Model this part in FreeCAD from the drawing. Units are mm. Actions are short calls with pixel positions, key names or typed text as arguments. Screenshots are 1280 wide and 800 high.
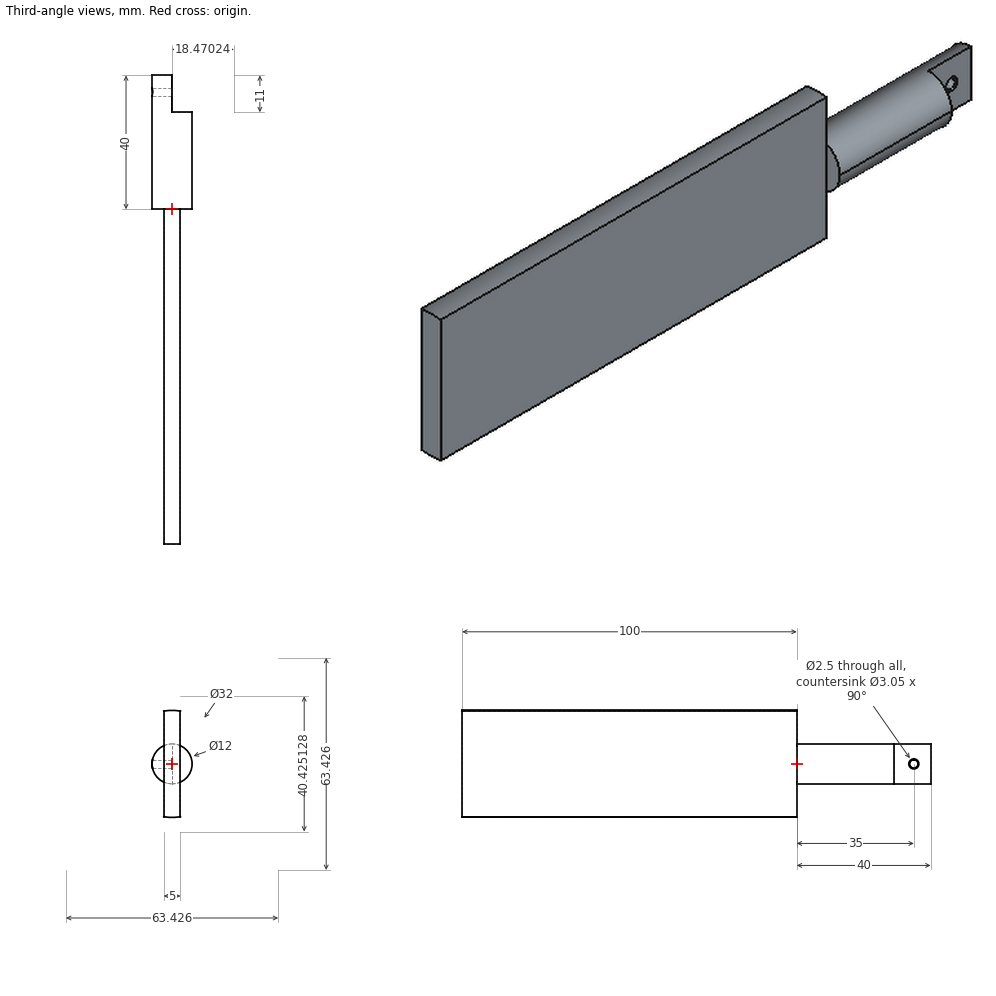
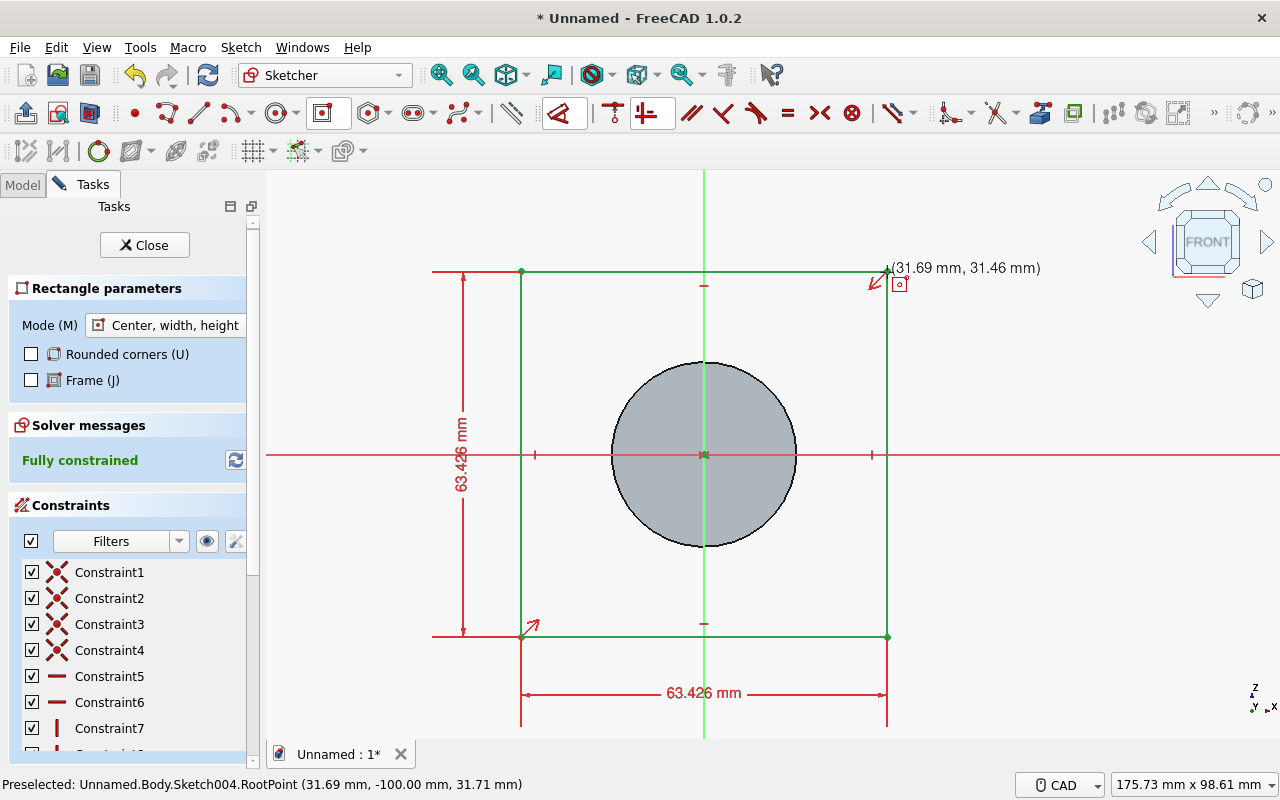
click(704, 454)
move(719, 338)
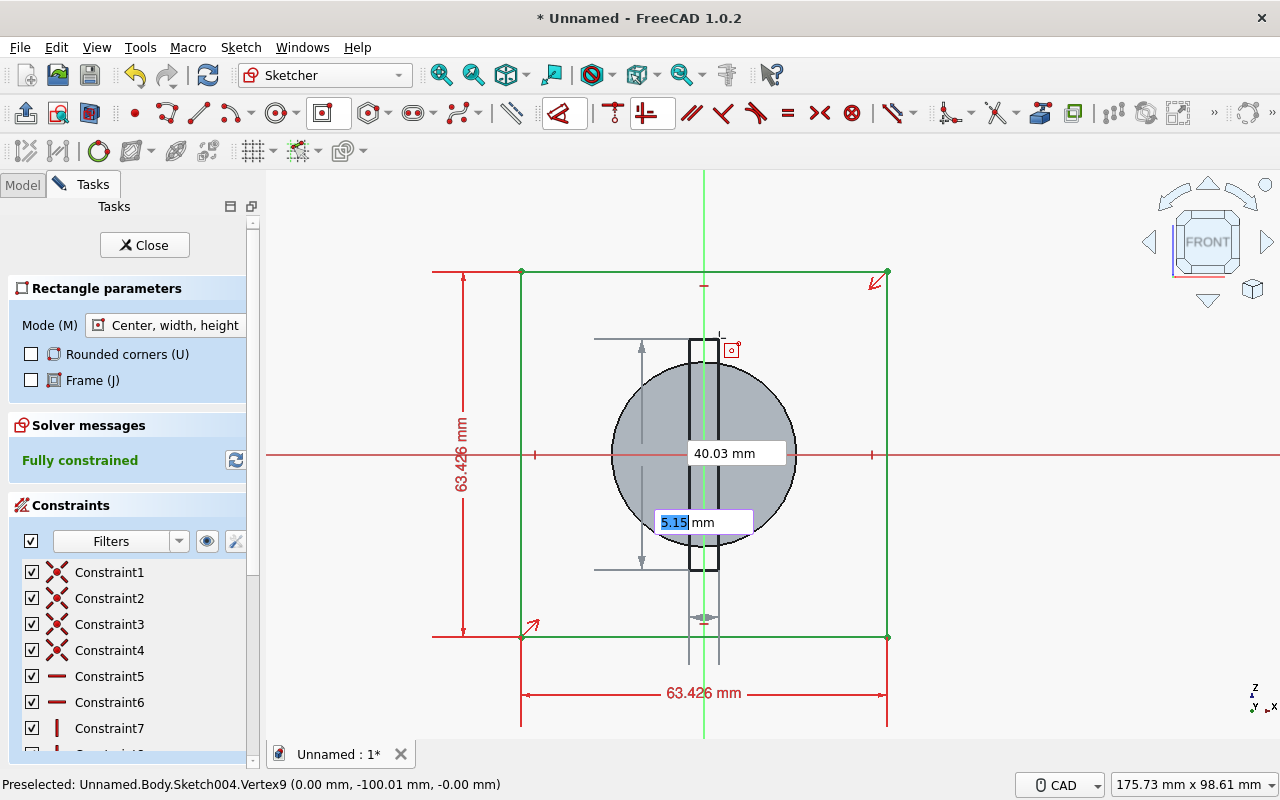
text(5)
key(Tab)
text(40.425128)
key(Return)
key(Escape)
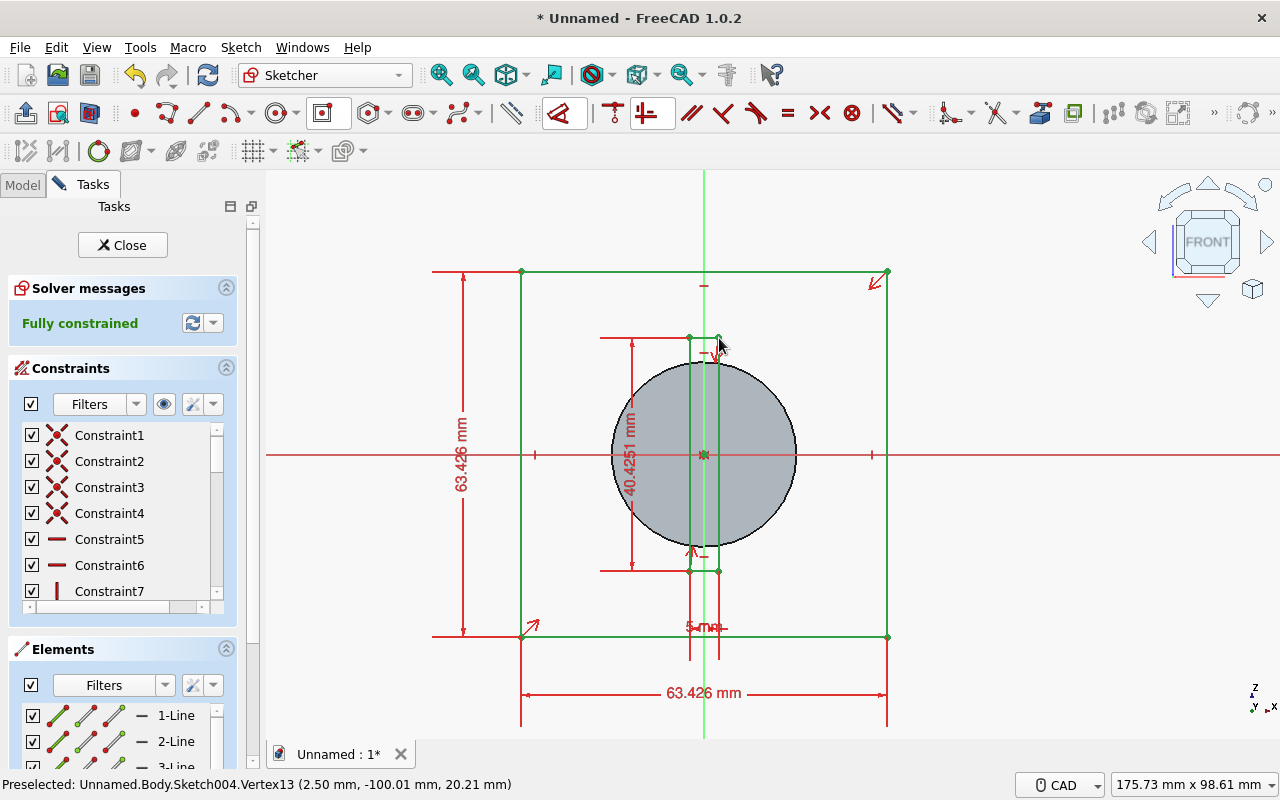
click(123, 245)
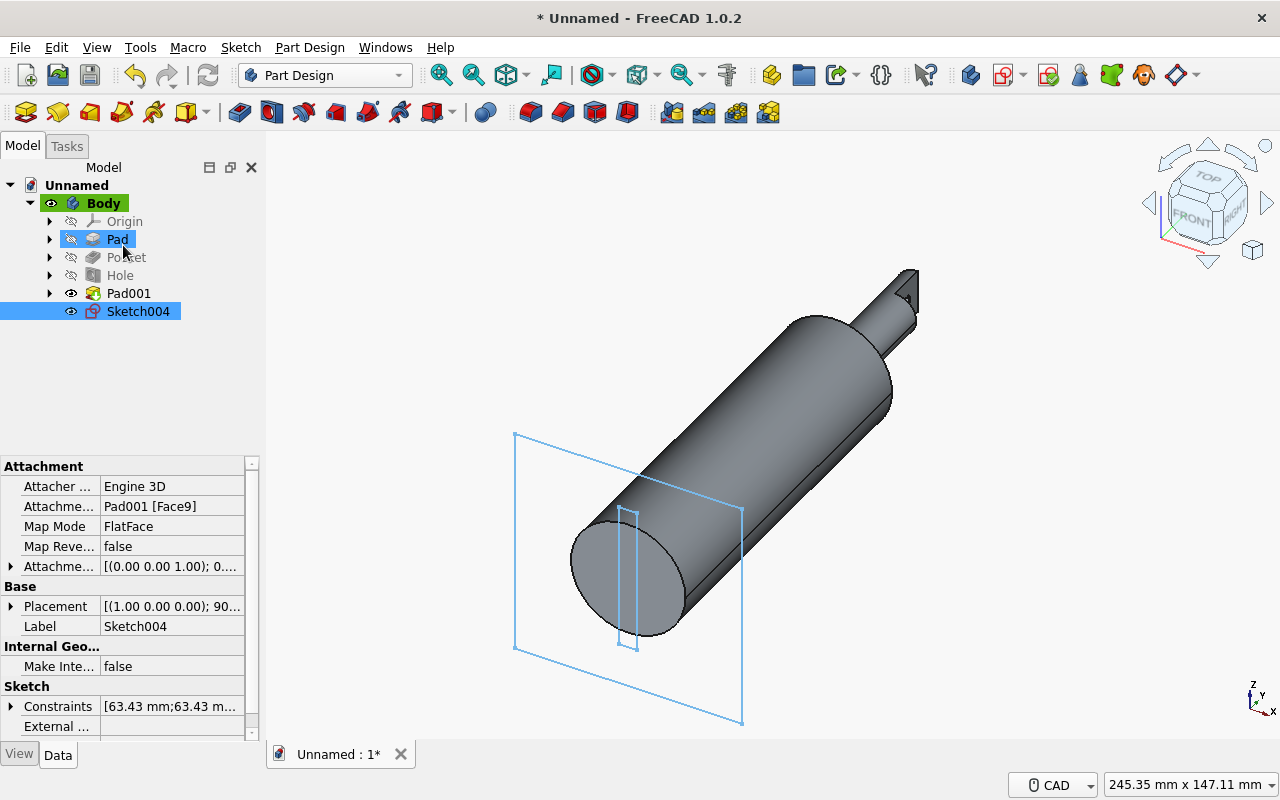
click(240, 112)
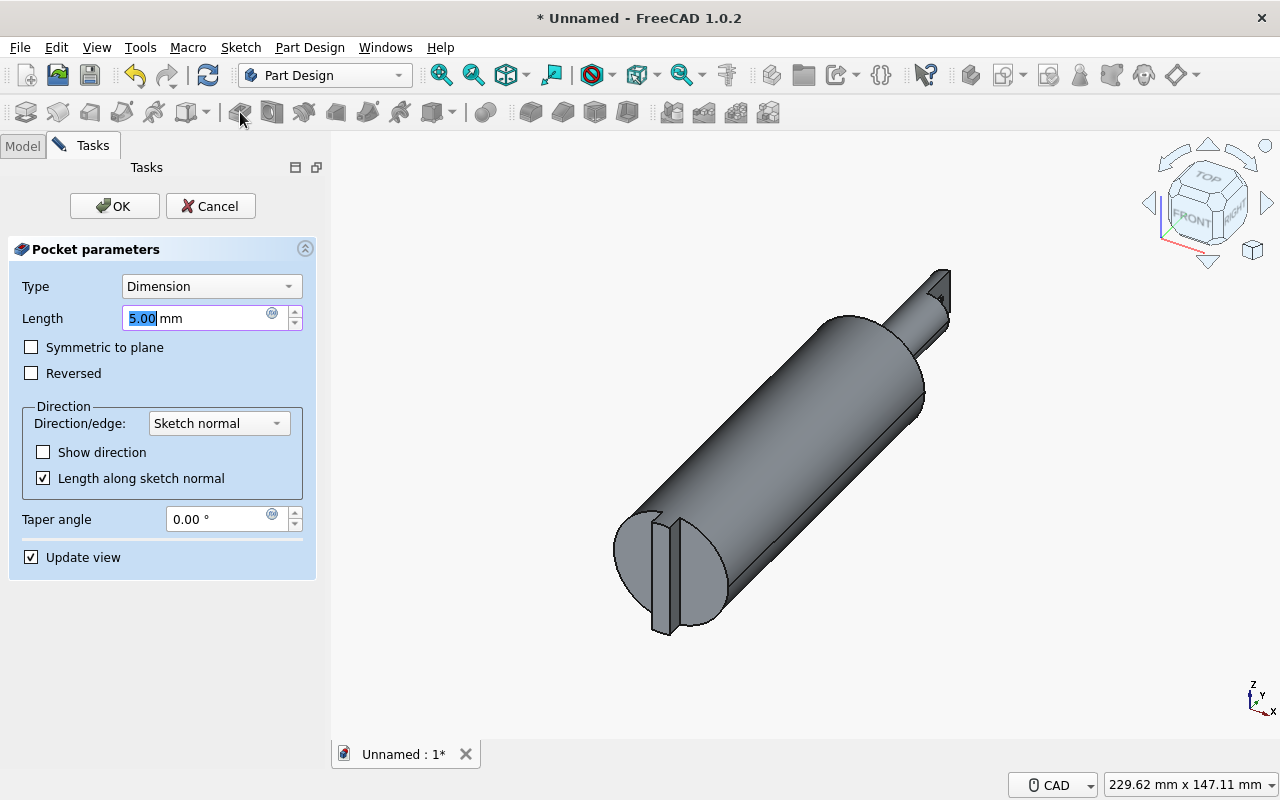
click(212, 286)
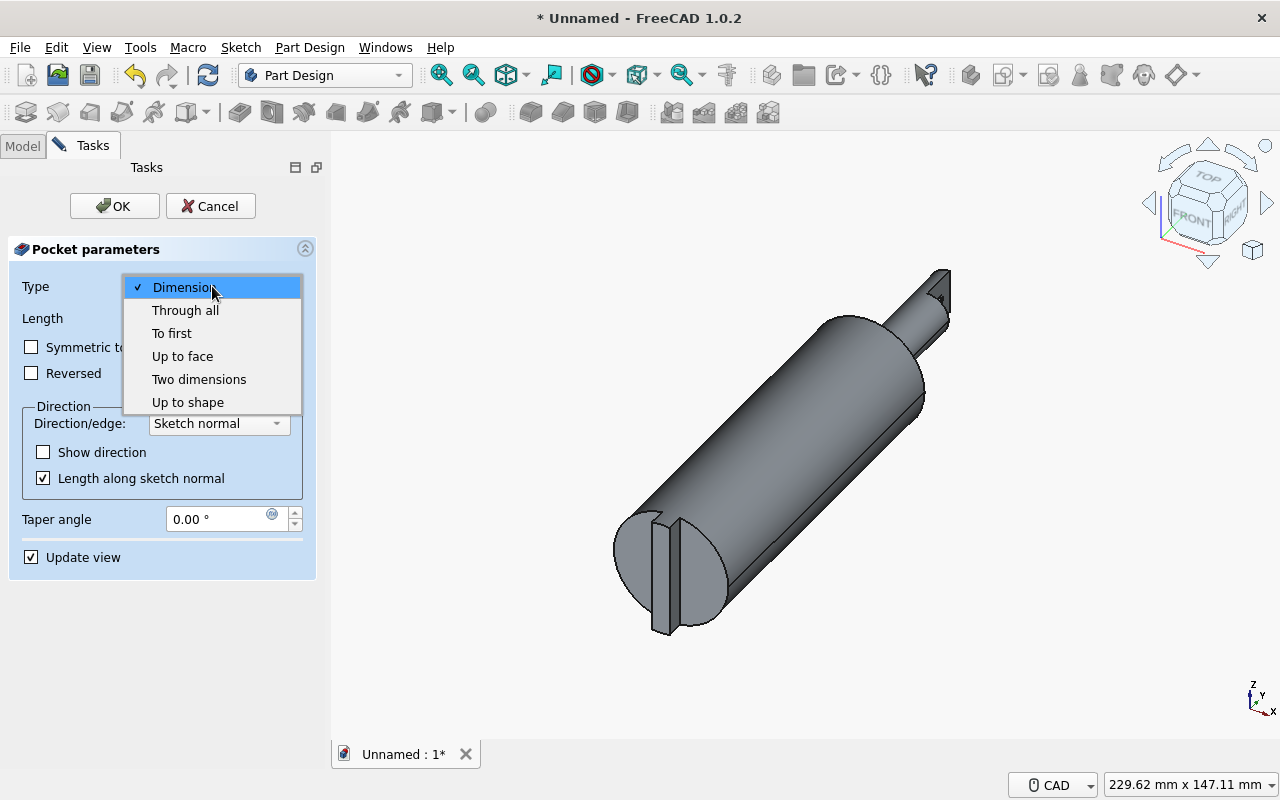
click(212, 380)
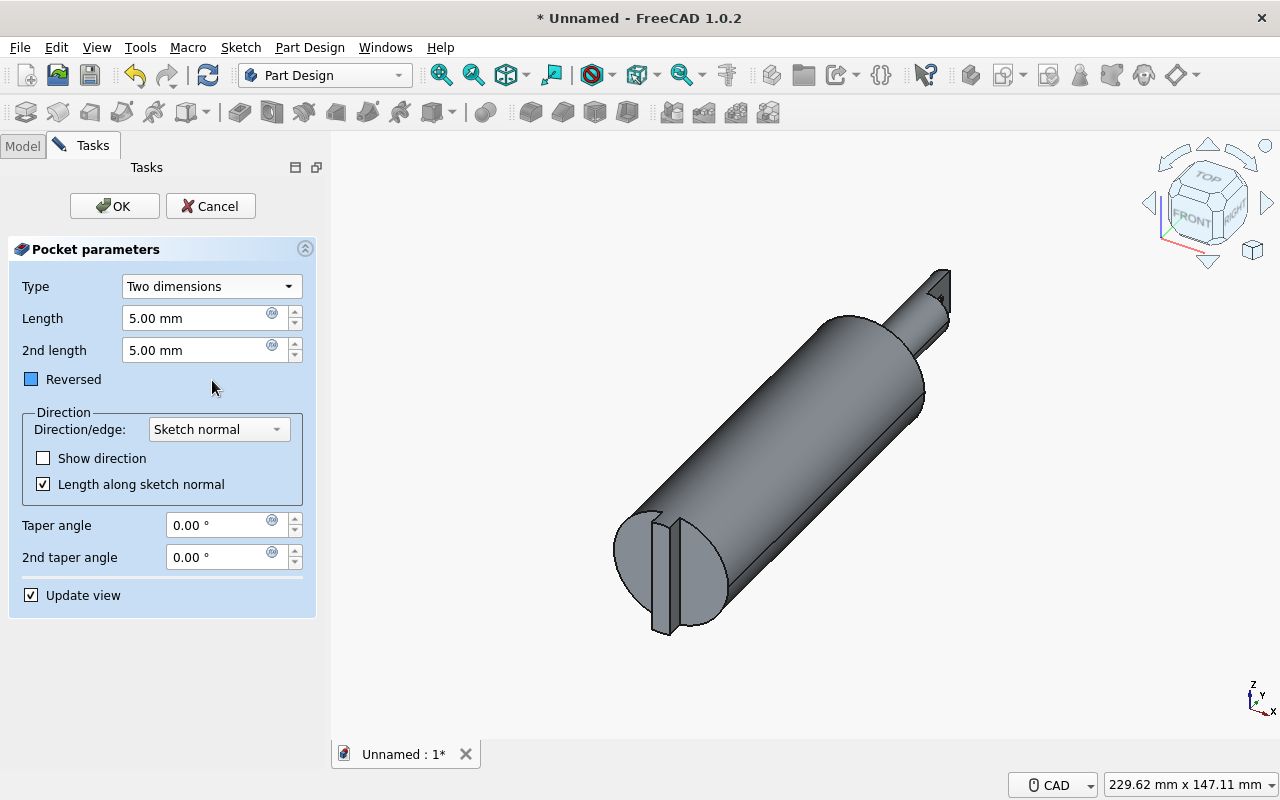
triple_click(204, 318)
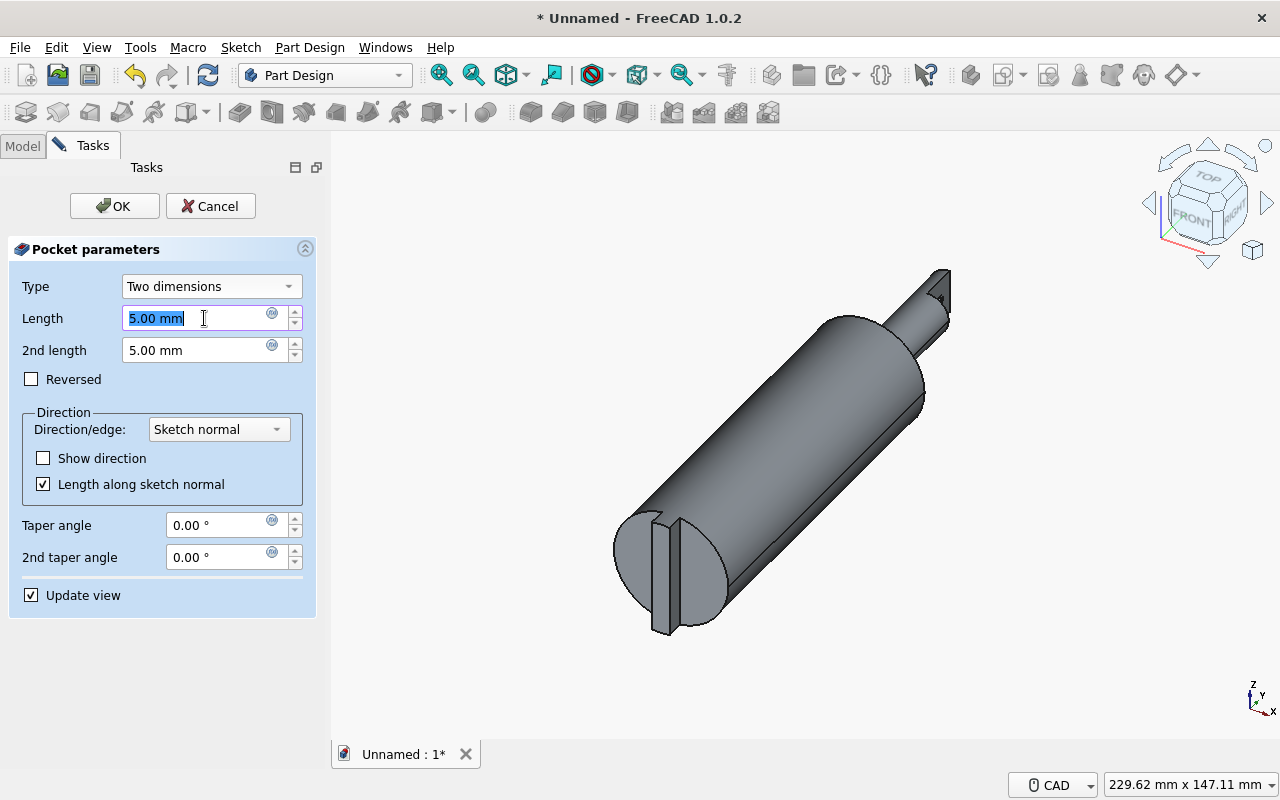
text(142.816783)
key(Tab)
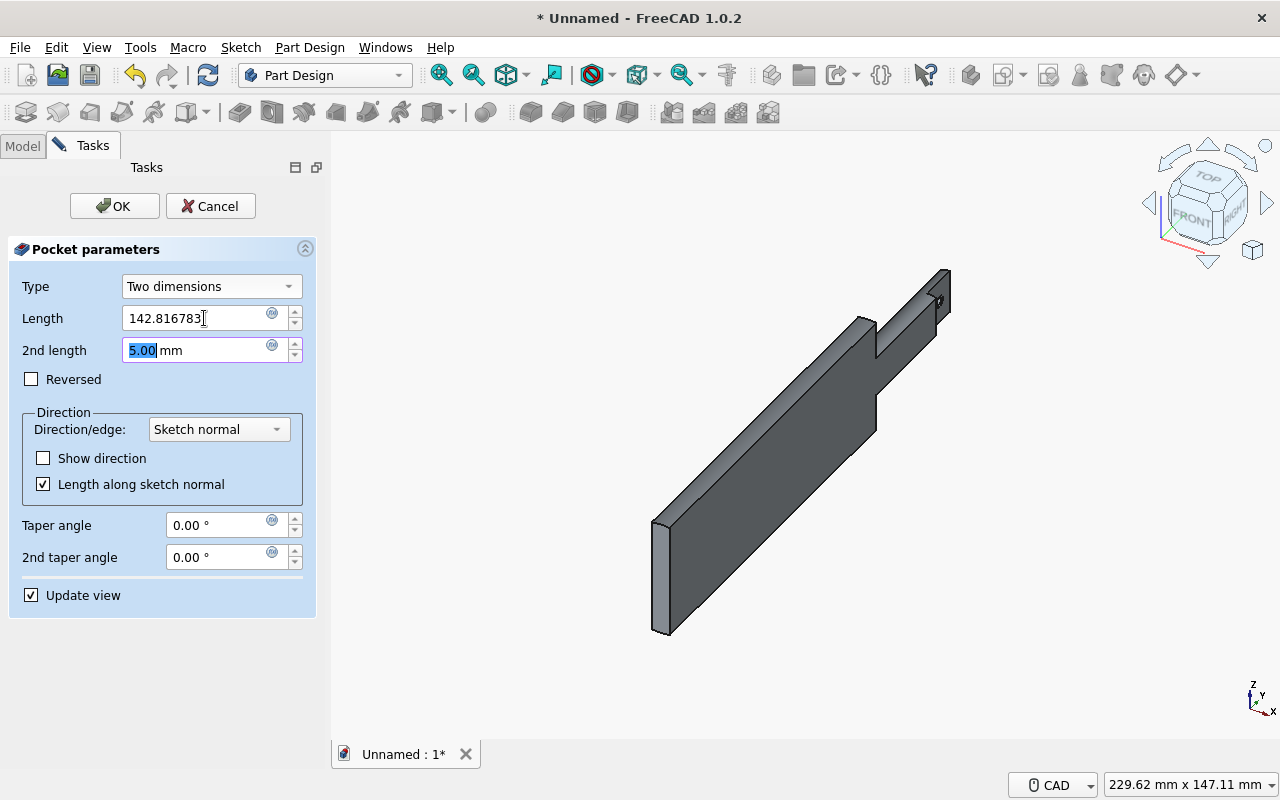
text(100)
key(Tab)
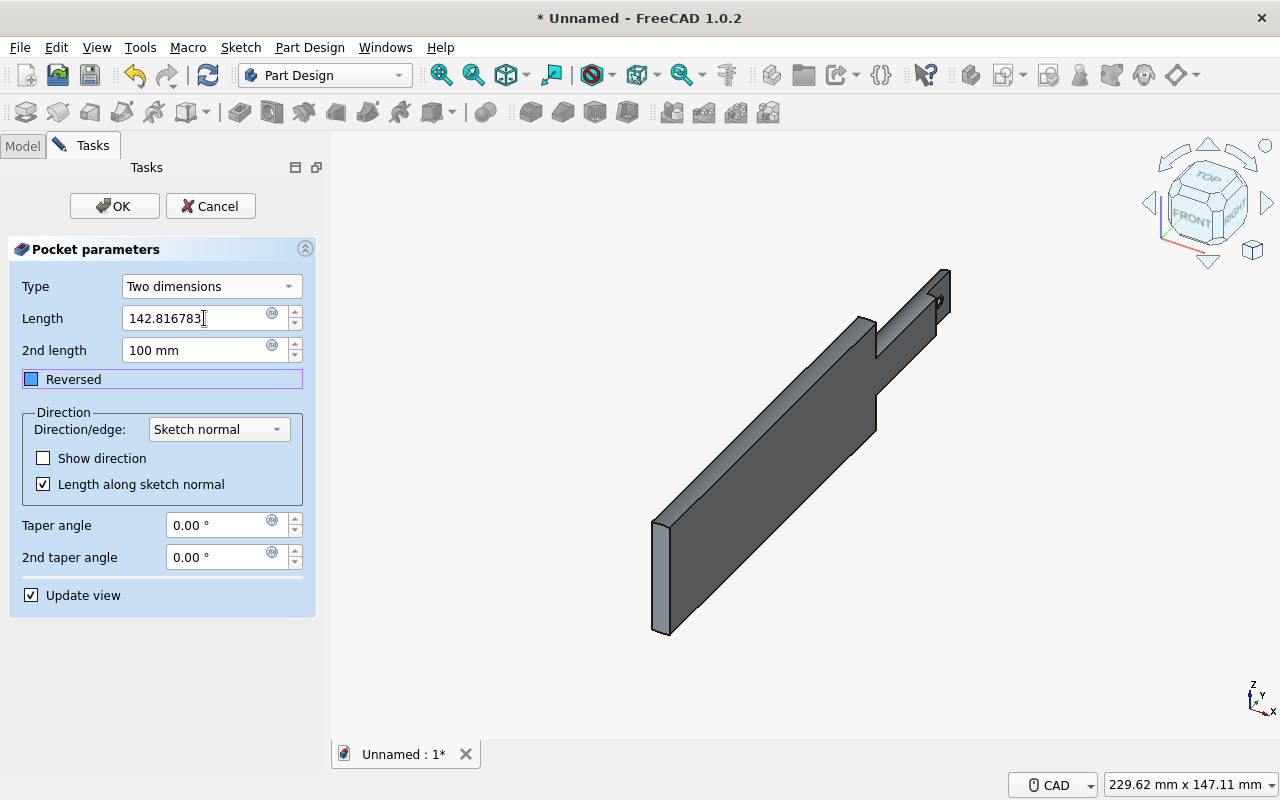
click(30, 379)